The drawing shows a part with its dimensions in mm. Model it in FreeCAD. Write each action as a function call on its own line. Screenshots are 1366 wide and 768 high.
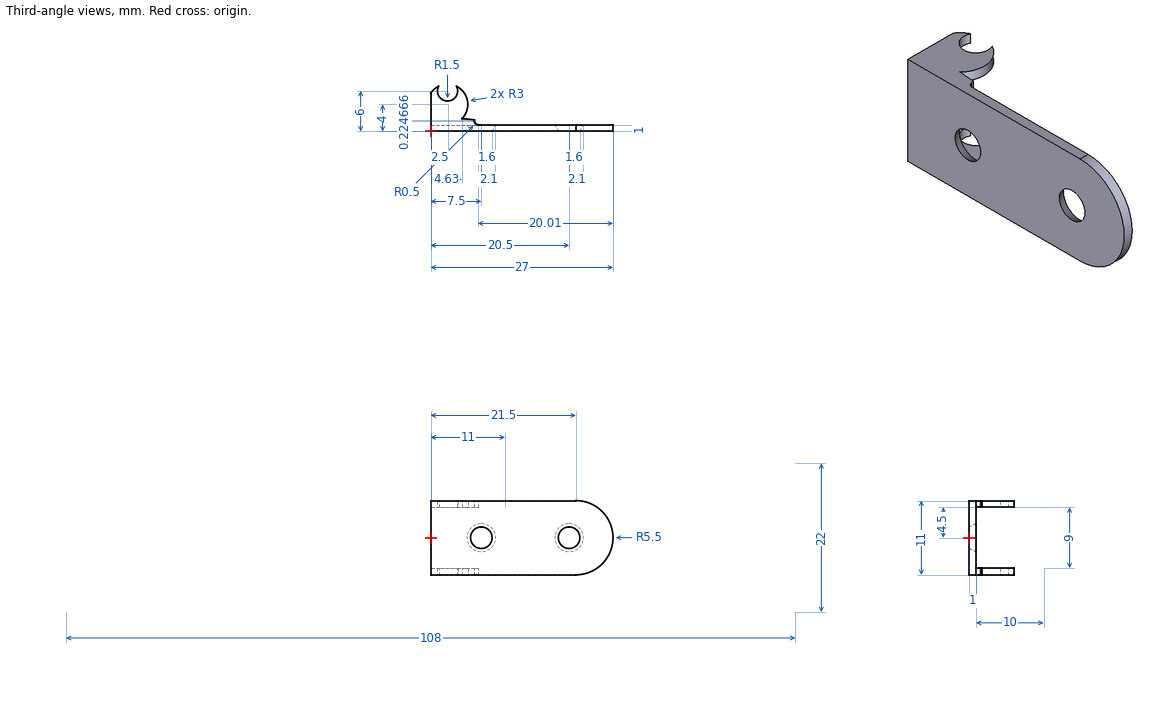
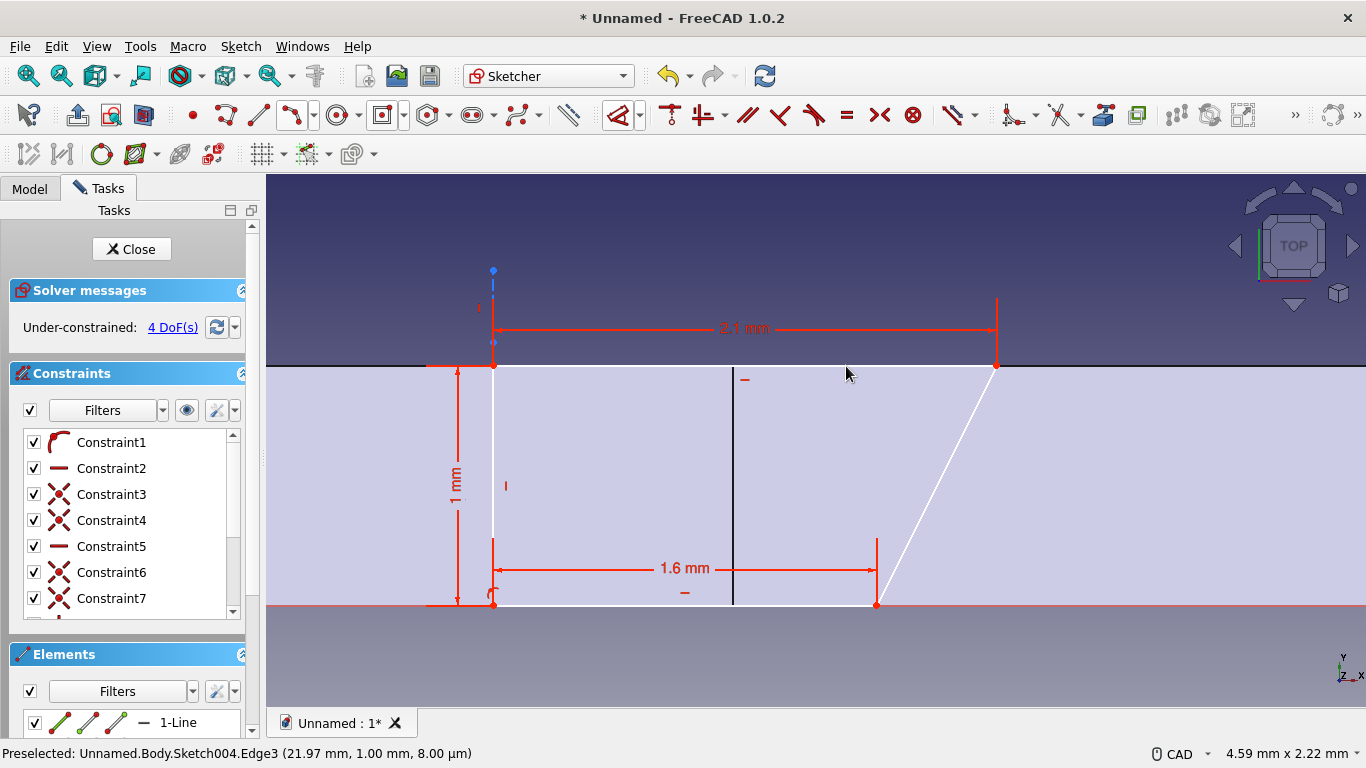
click(493, 606)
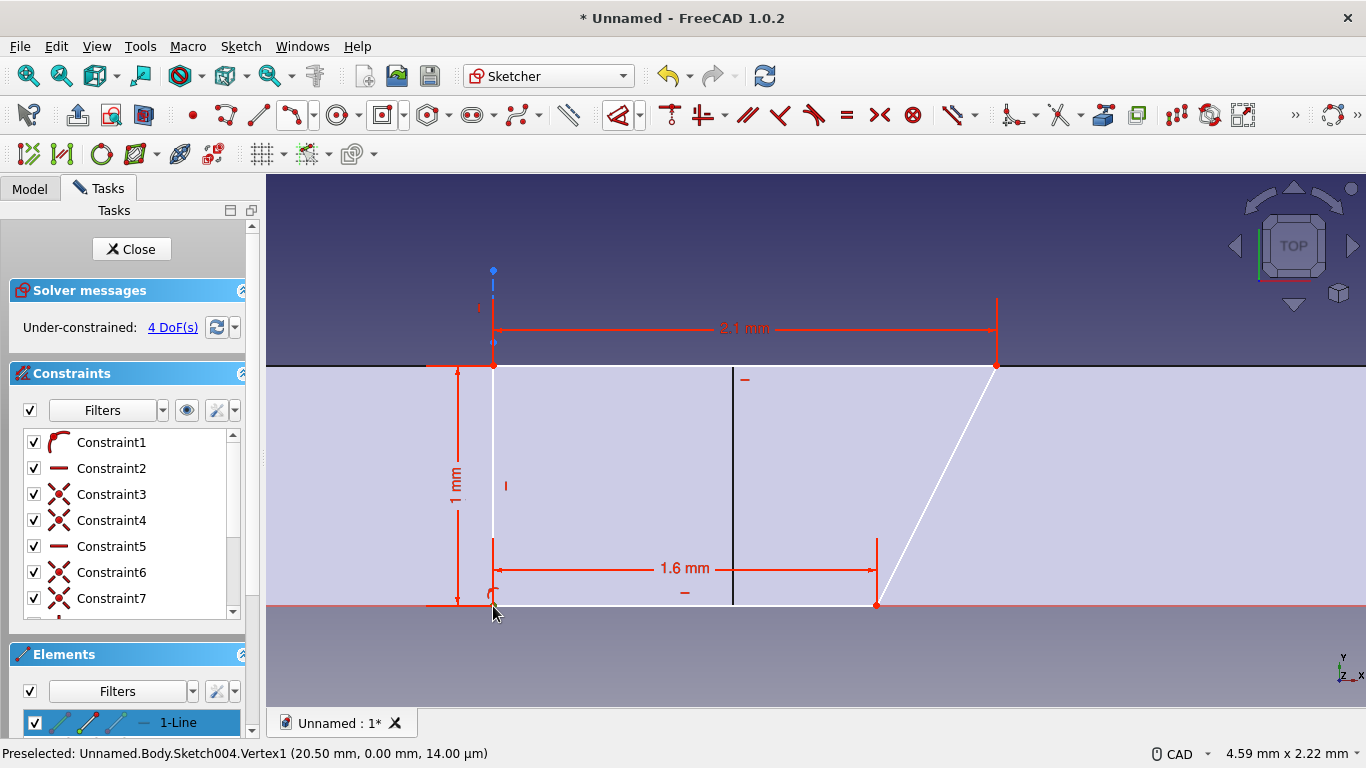
key(l)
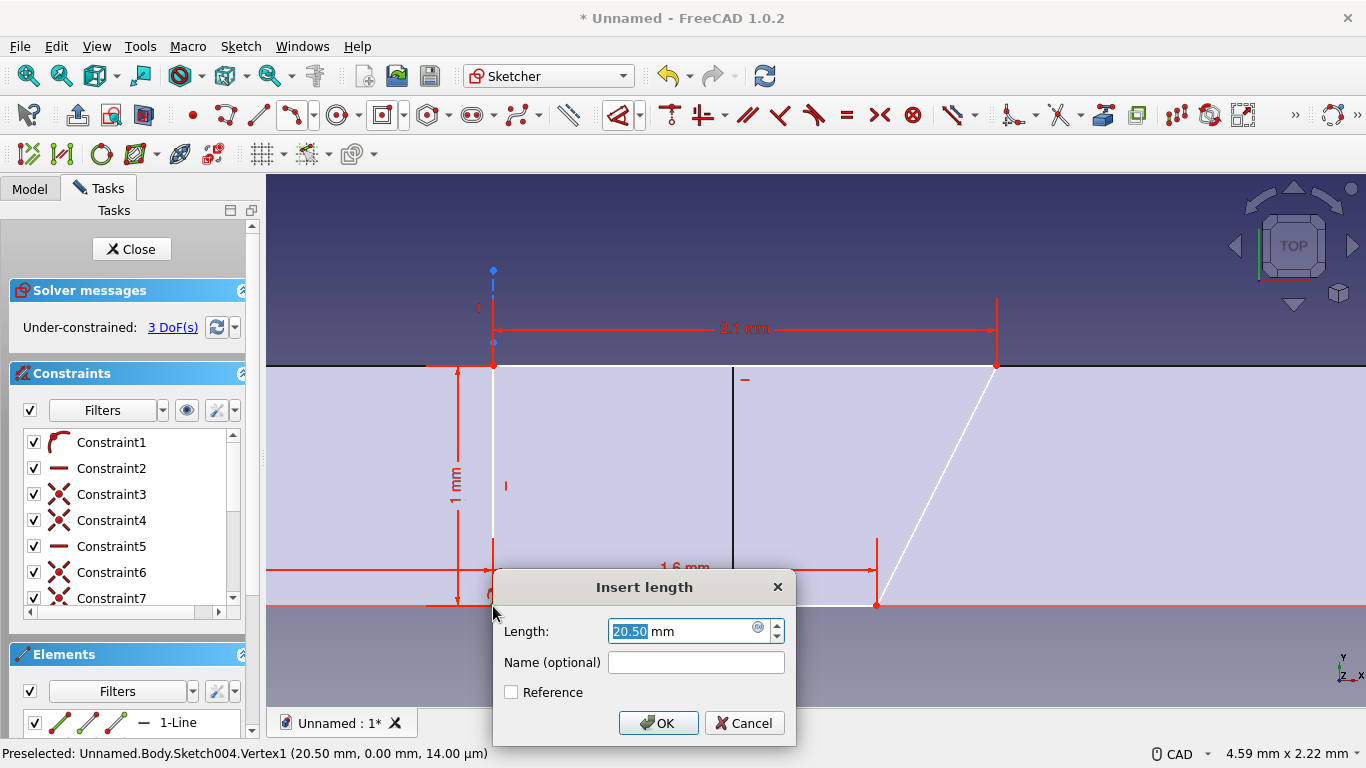
text(20.5)
key(Return)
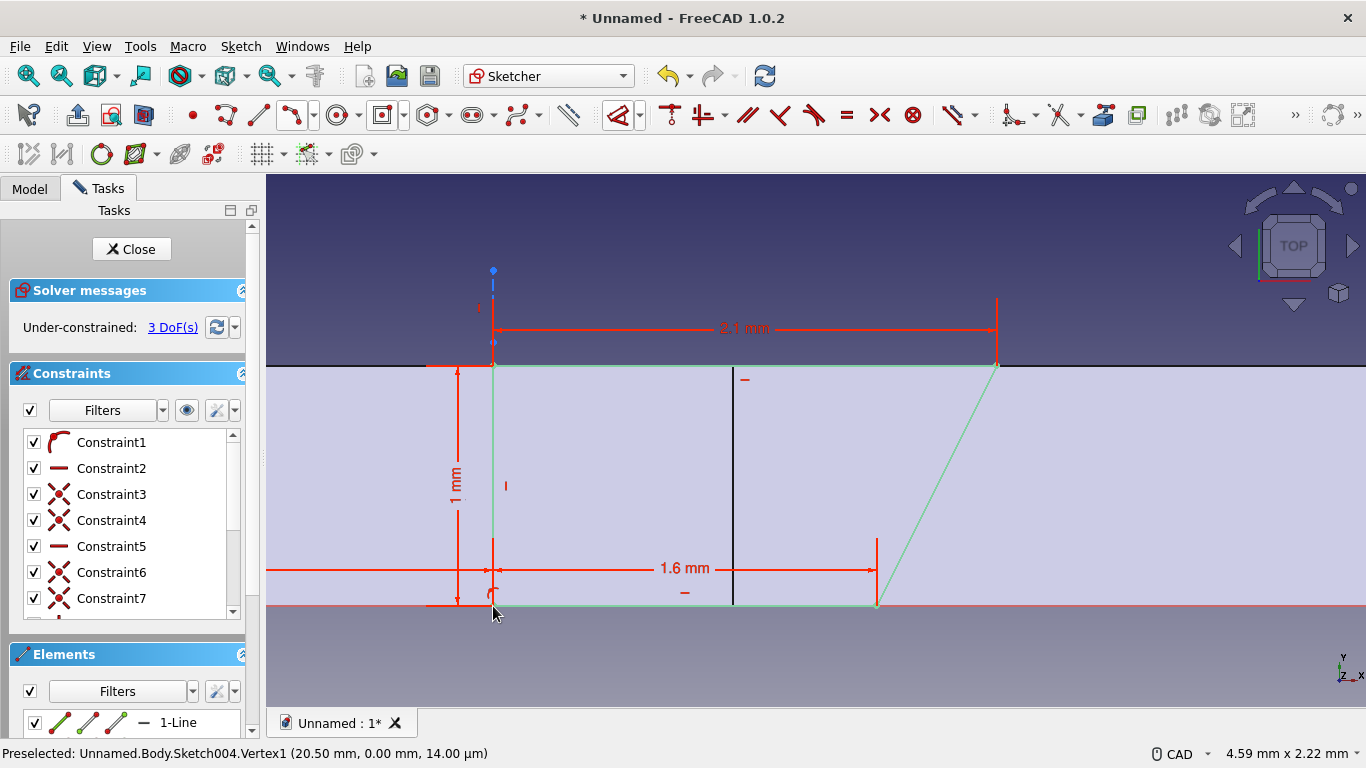
click(493, 343)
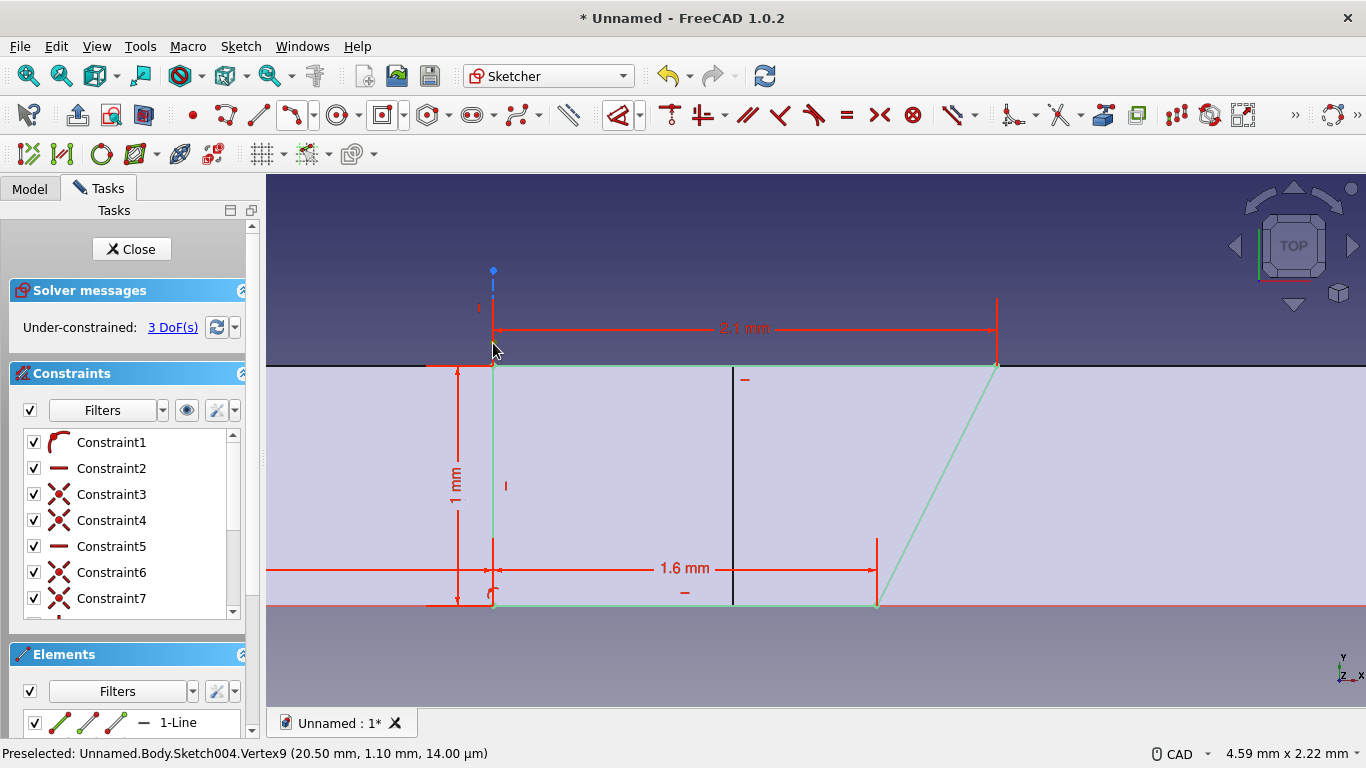
key(l)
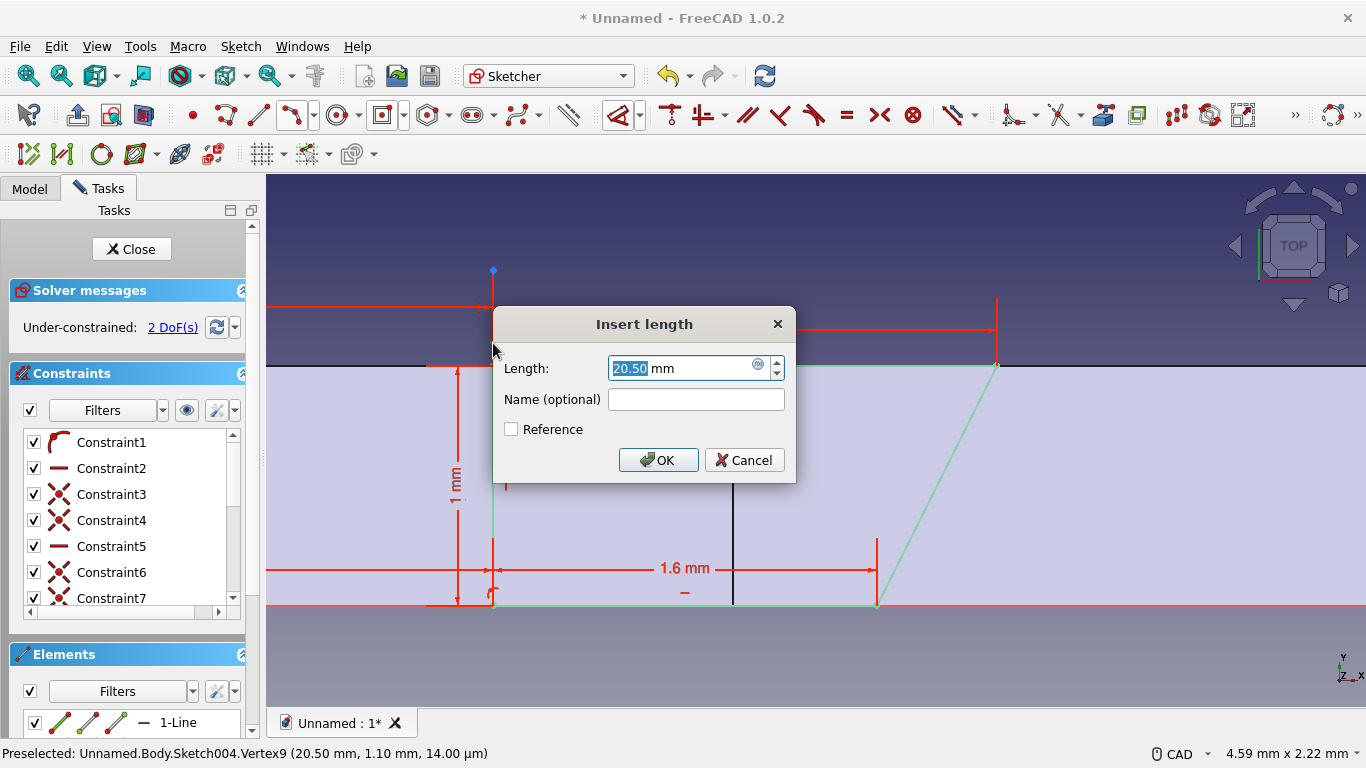
text(20.5)
key(Return)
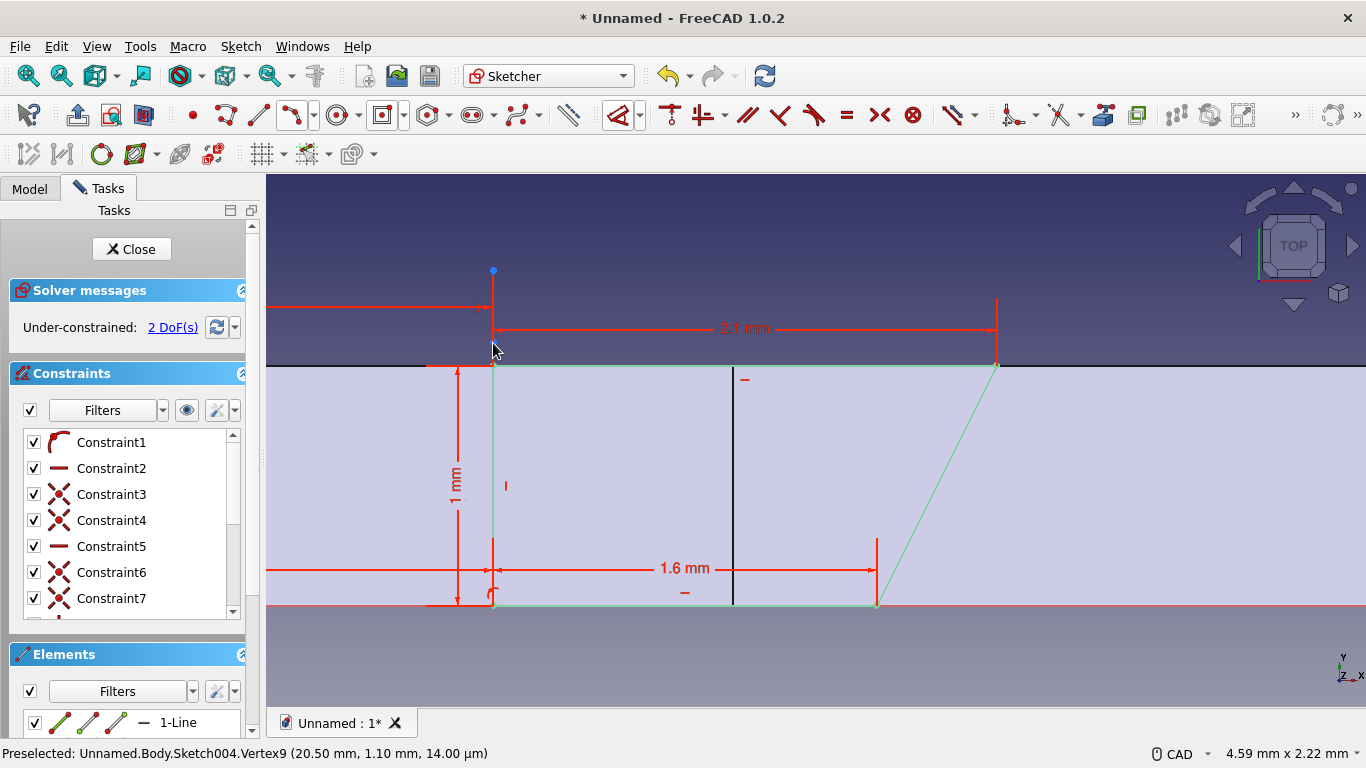
click(132, 249)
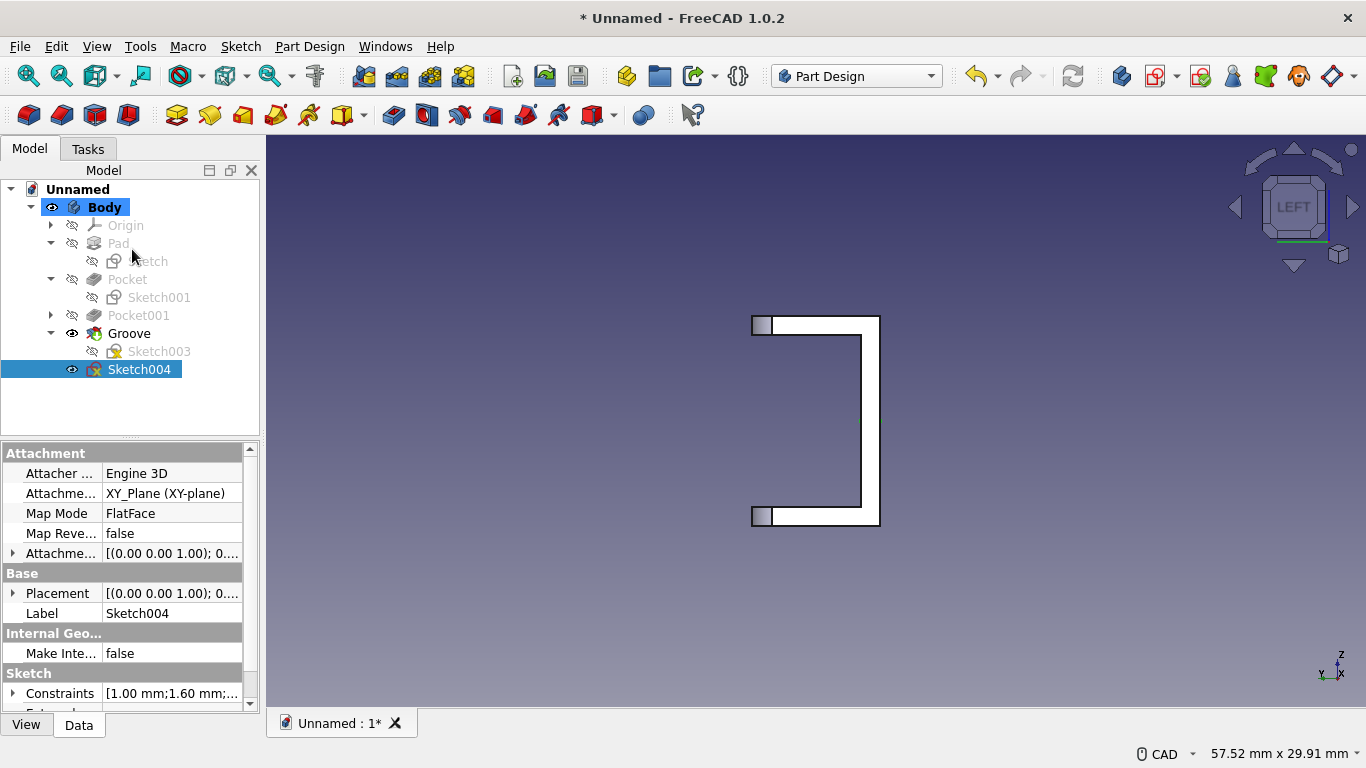
click(460, 116)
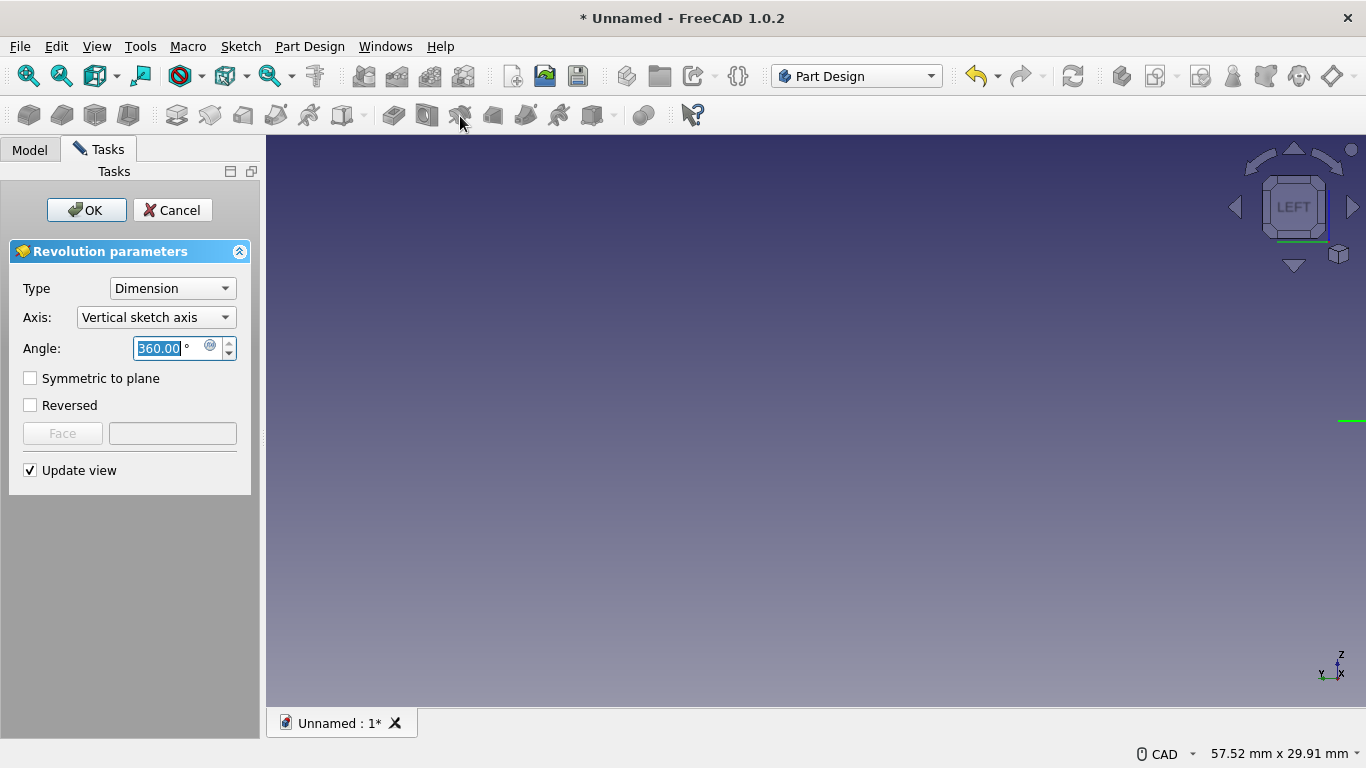
click(157, 318)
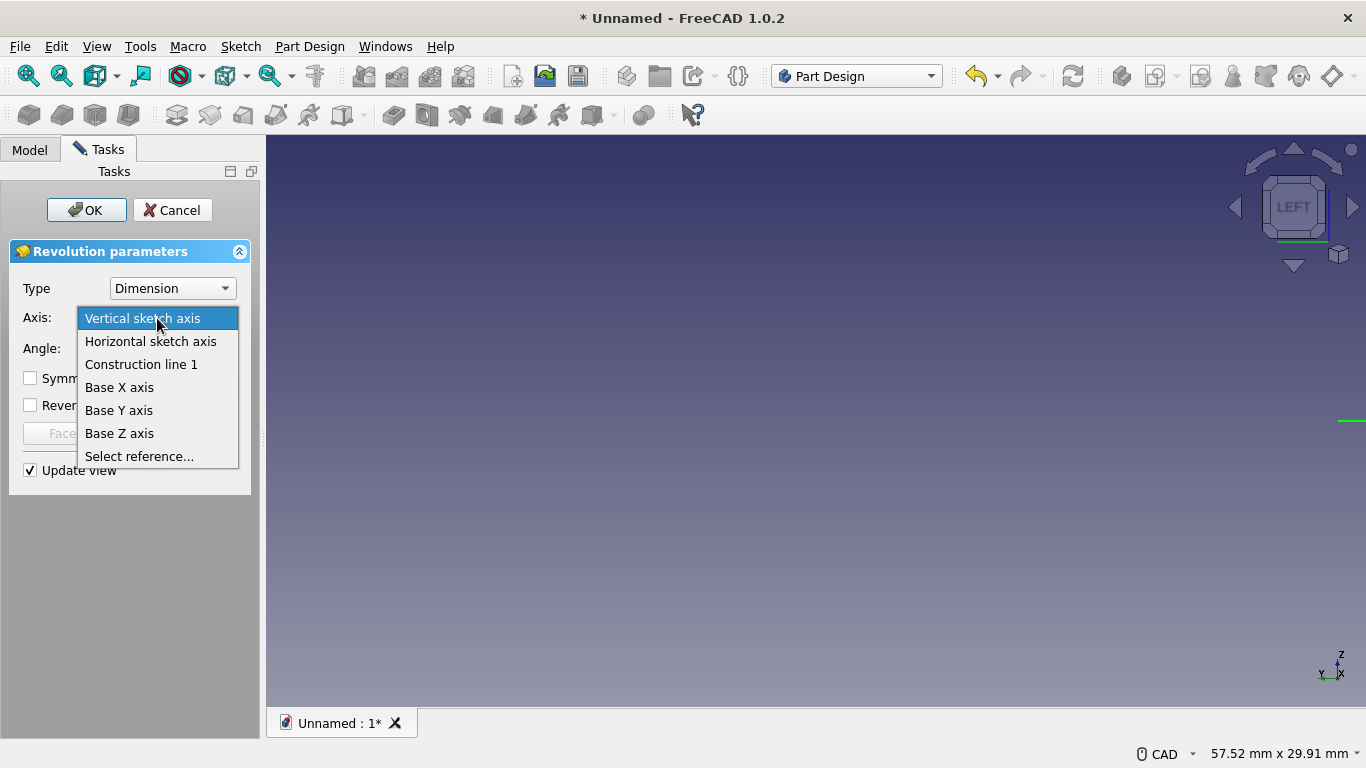
click(156, 364)